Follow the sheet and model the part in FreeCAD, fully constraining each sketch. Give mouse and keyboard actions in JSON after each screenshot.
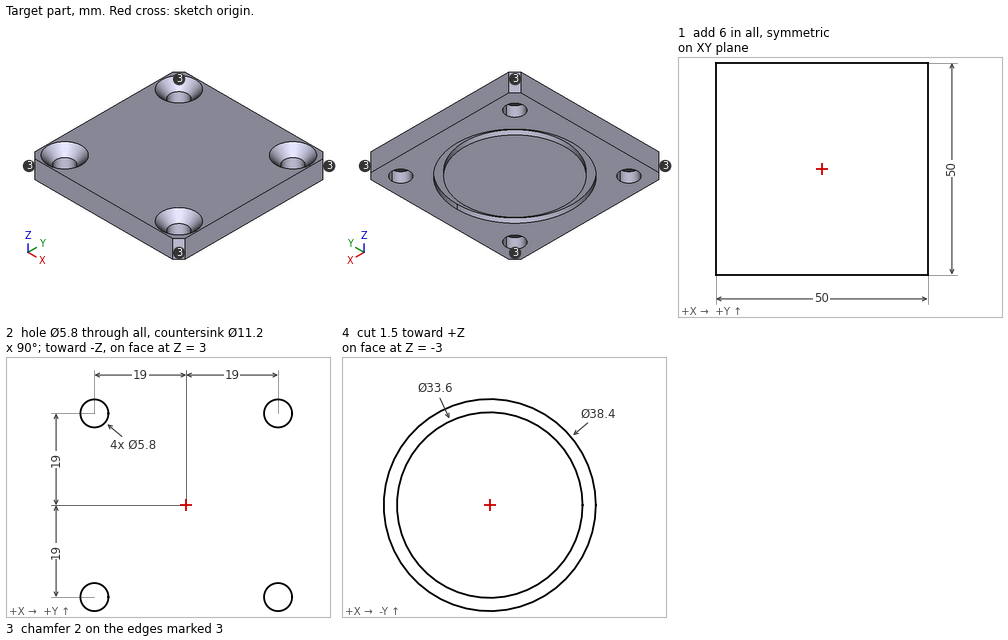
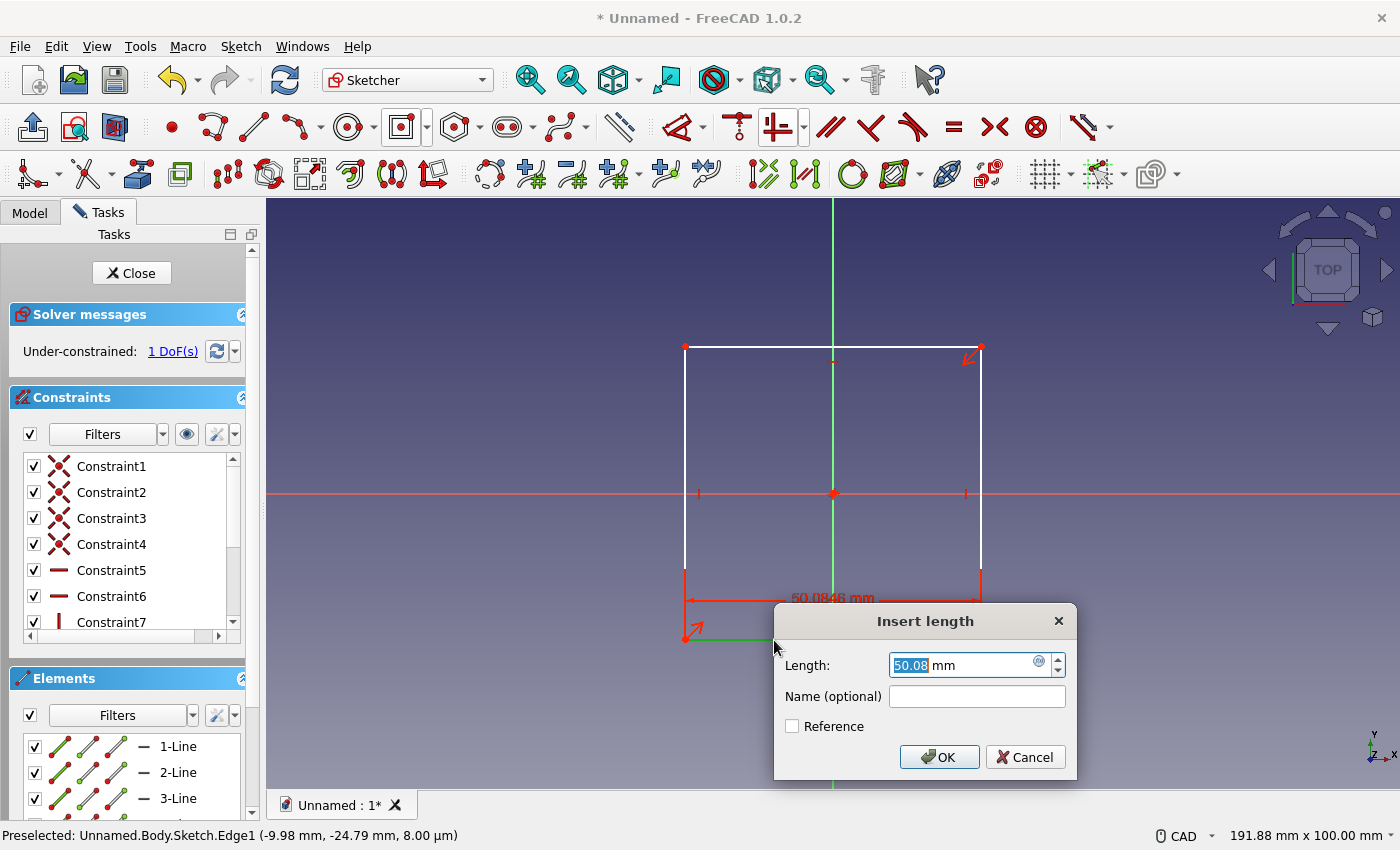
{"action": "type", "text": "50"}
{"action": "key", "text": "Return"}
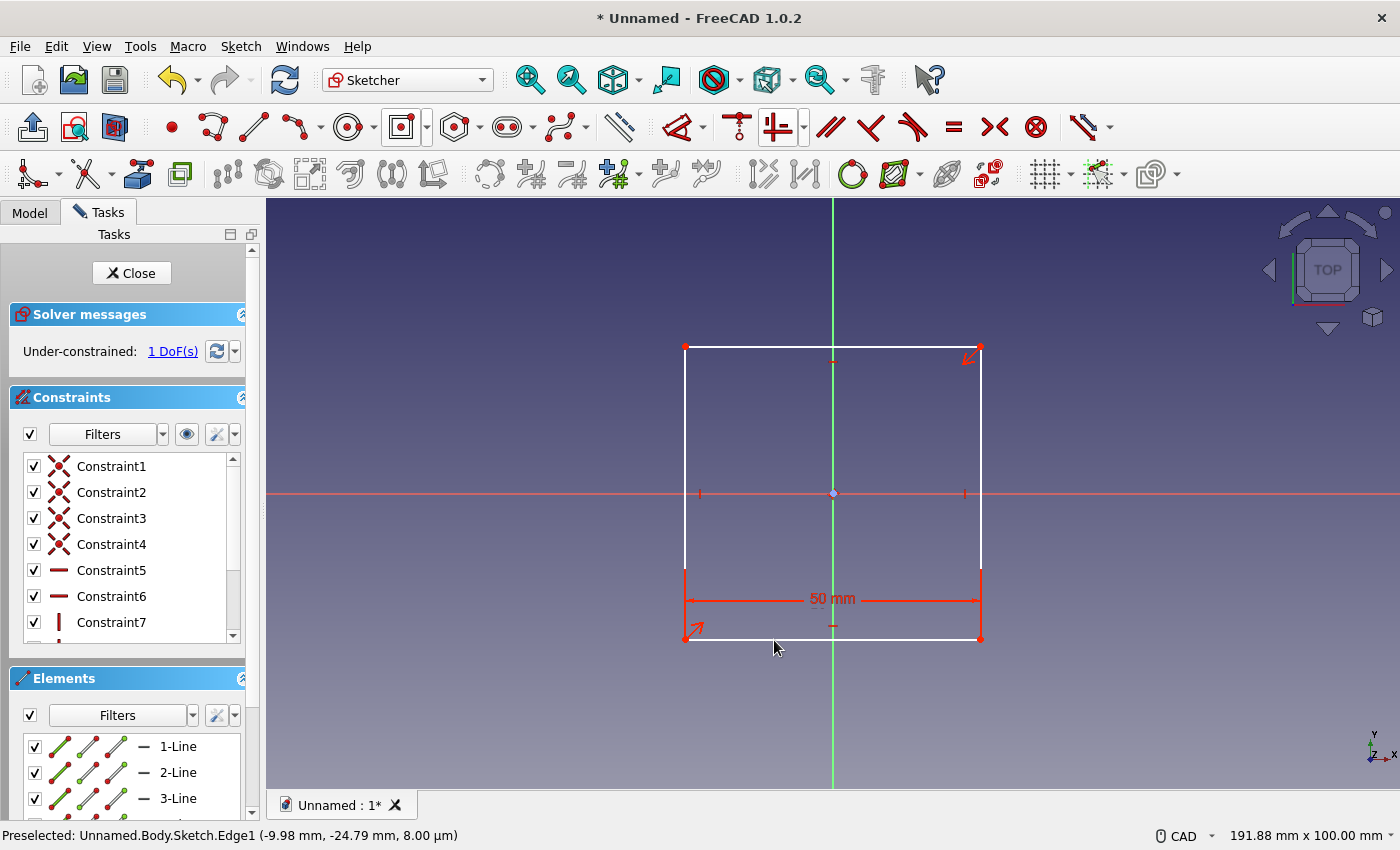
{"action": "left_click", "coordinate": [981, 552]}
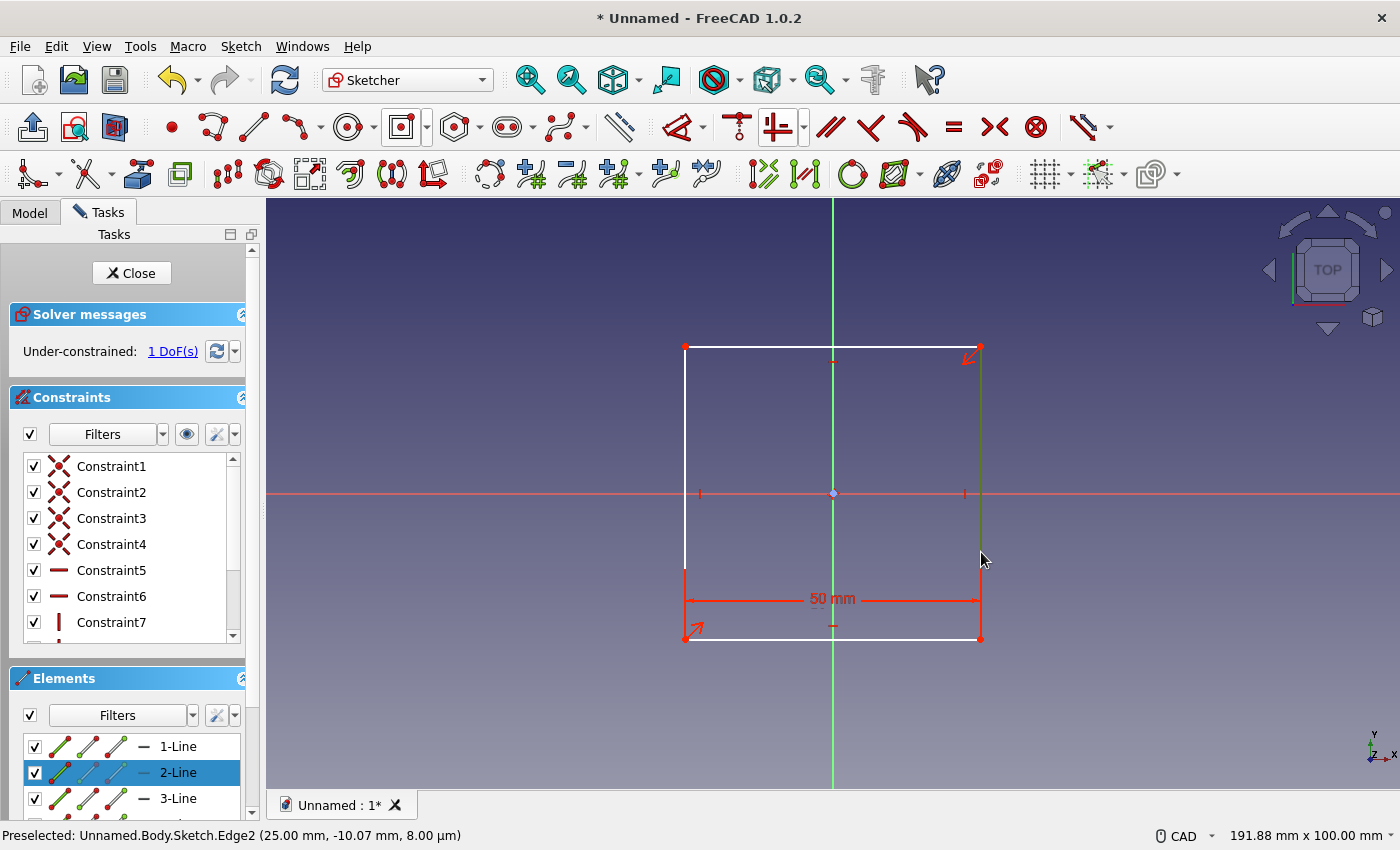
{"action": "left_click", "coordinate": [702, 128]}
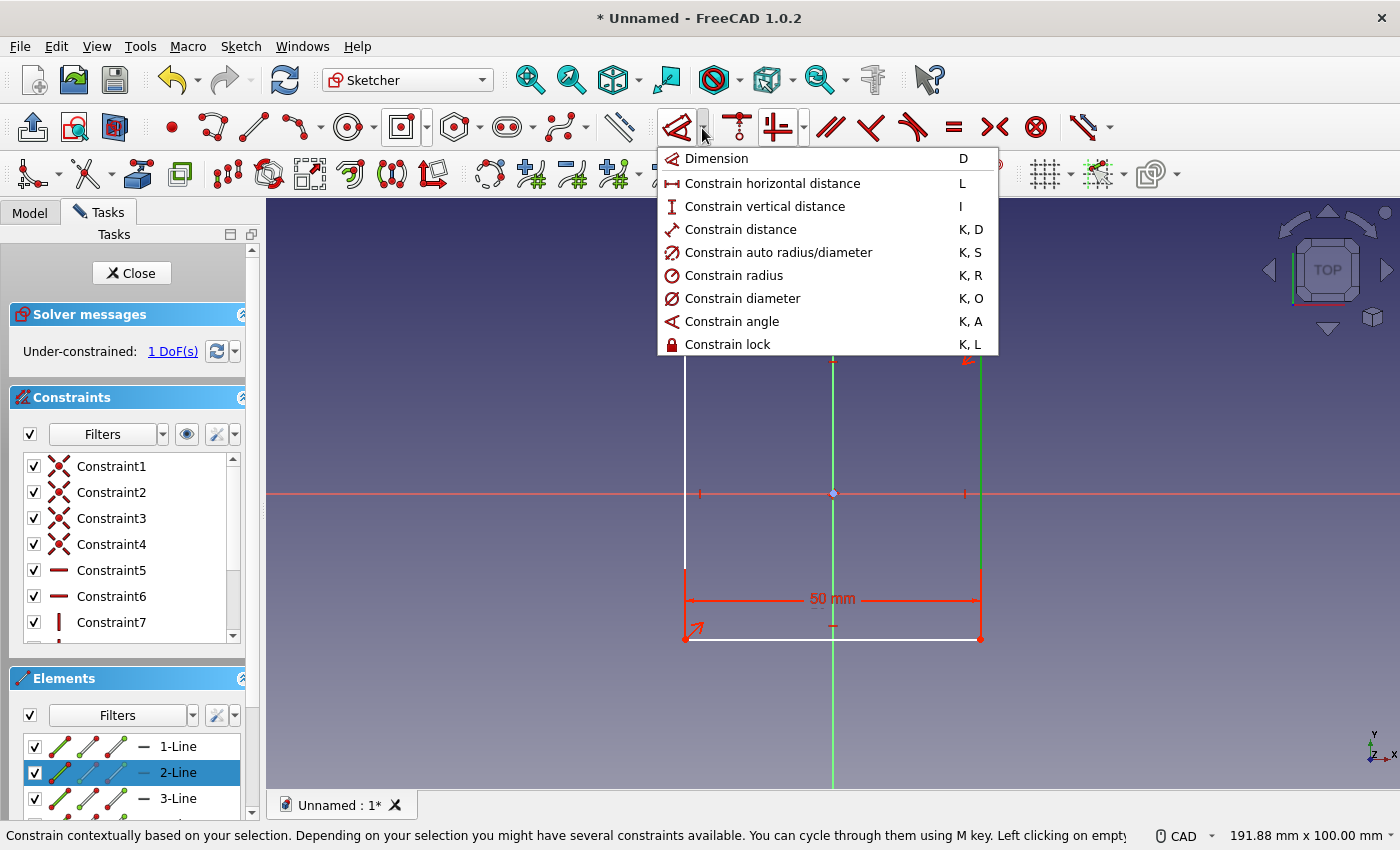
{"action": "left_click", "coordinate": [828, 206]}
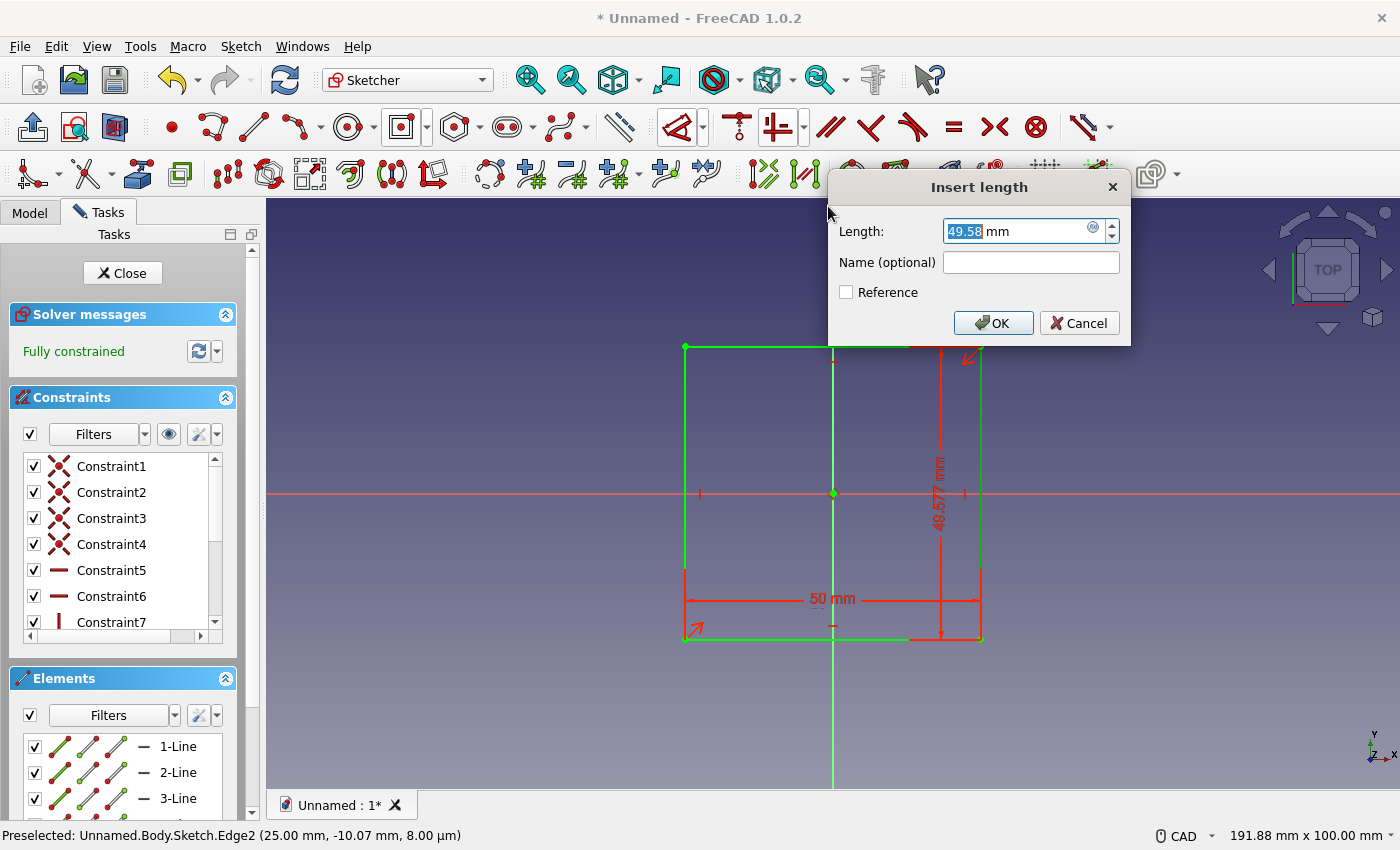
{"action": "type", "text": "50"}
{"action": "key", "text": "Return"}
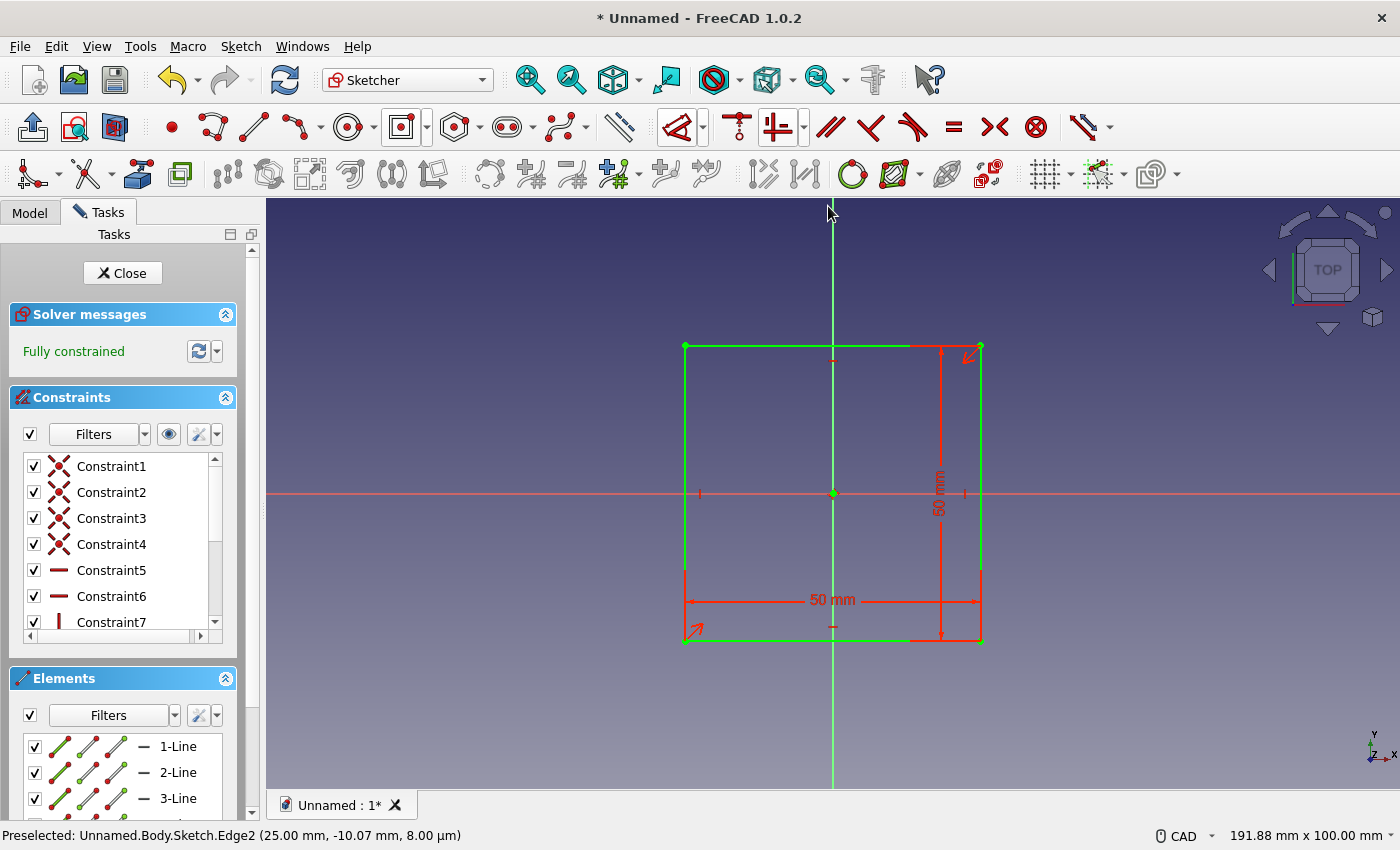
{"action": "left_click", "coordinate": [123, 273]}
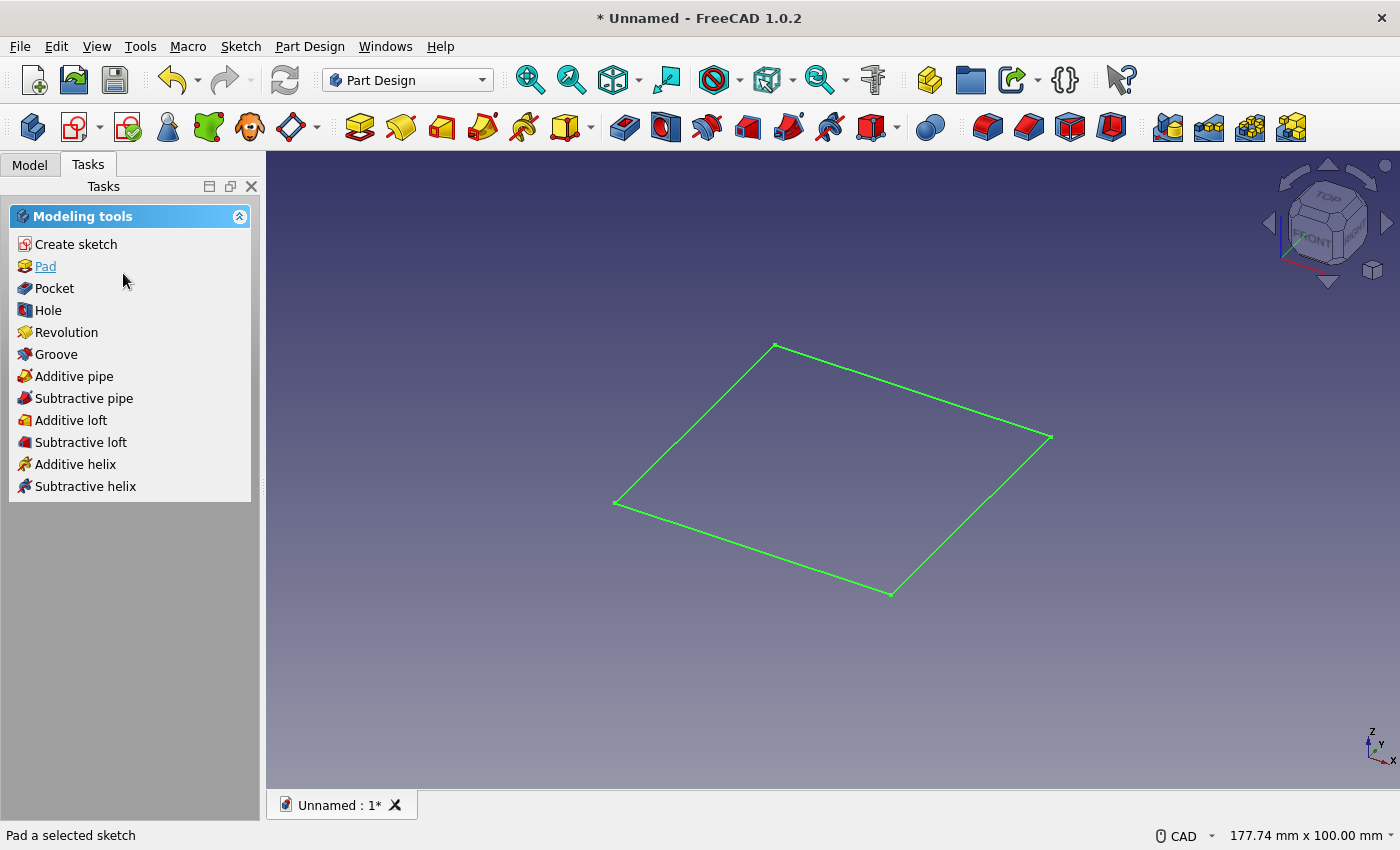
{"action": "left_click", "coordinate": [360, 128]}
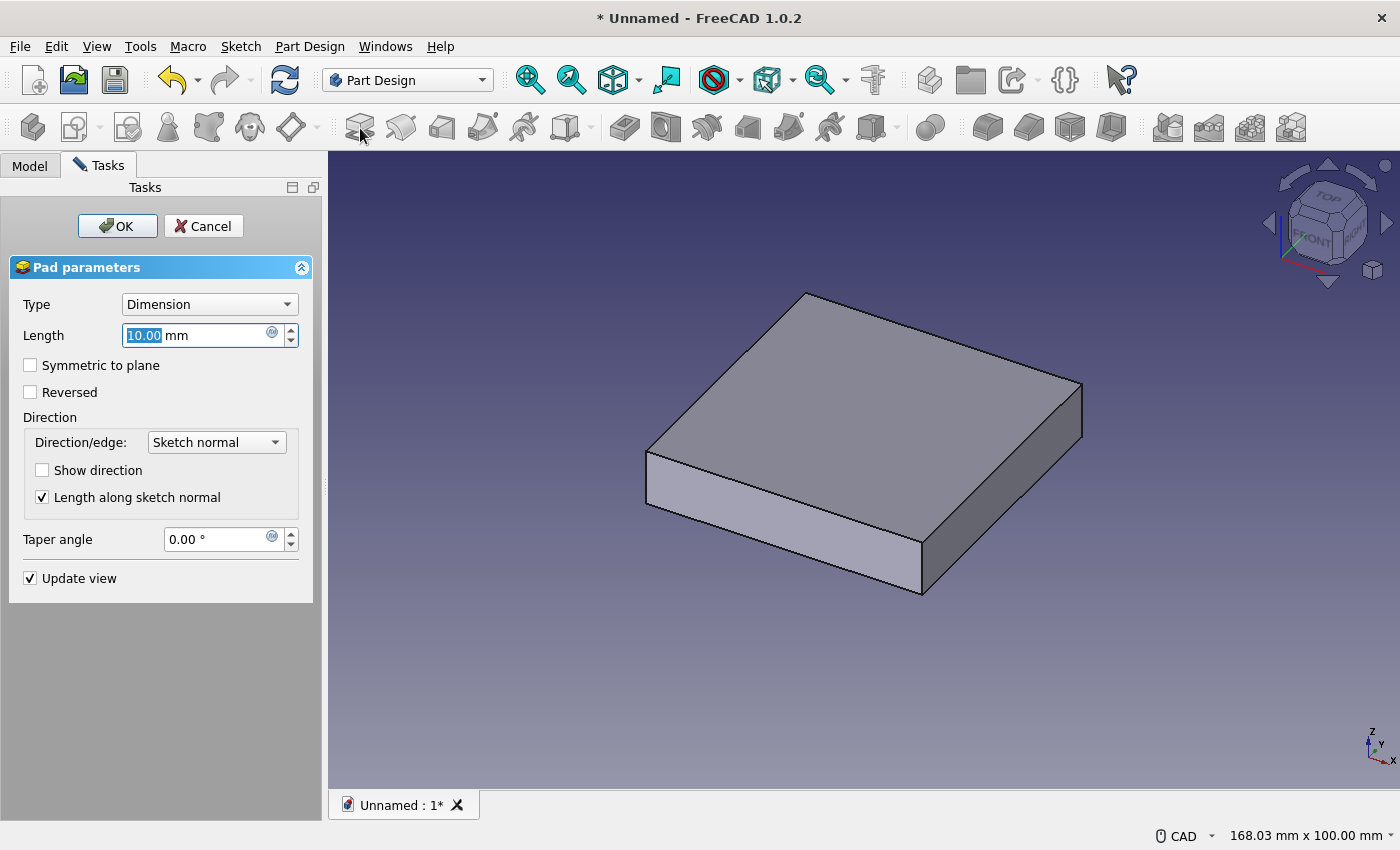
{"action": "type", "text": "6"}
{"action": "key", "text": "Tab"}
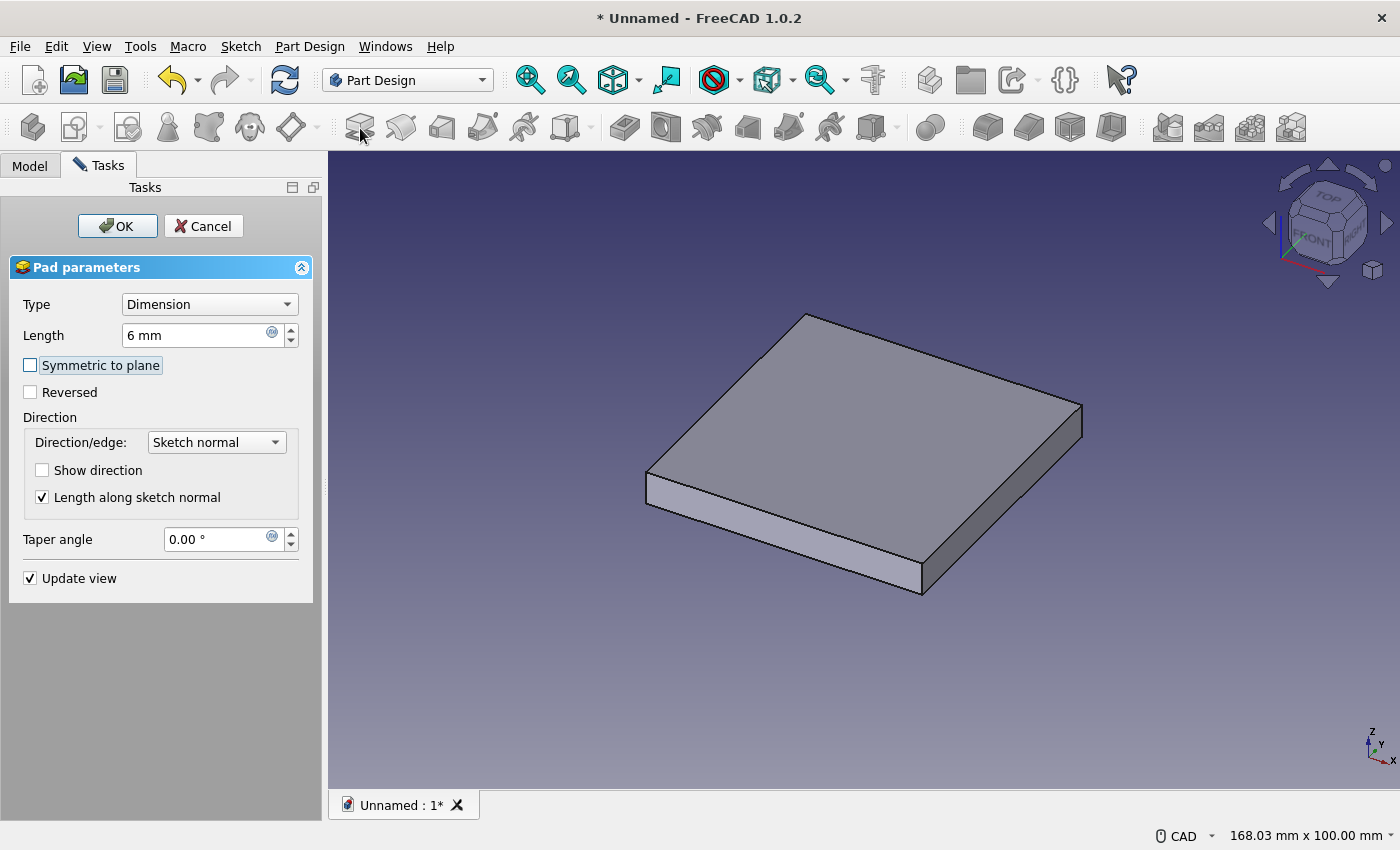
{"action": "left_click", "coordinate": [31, 365]}